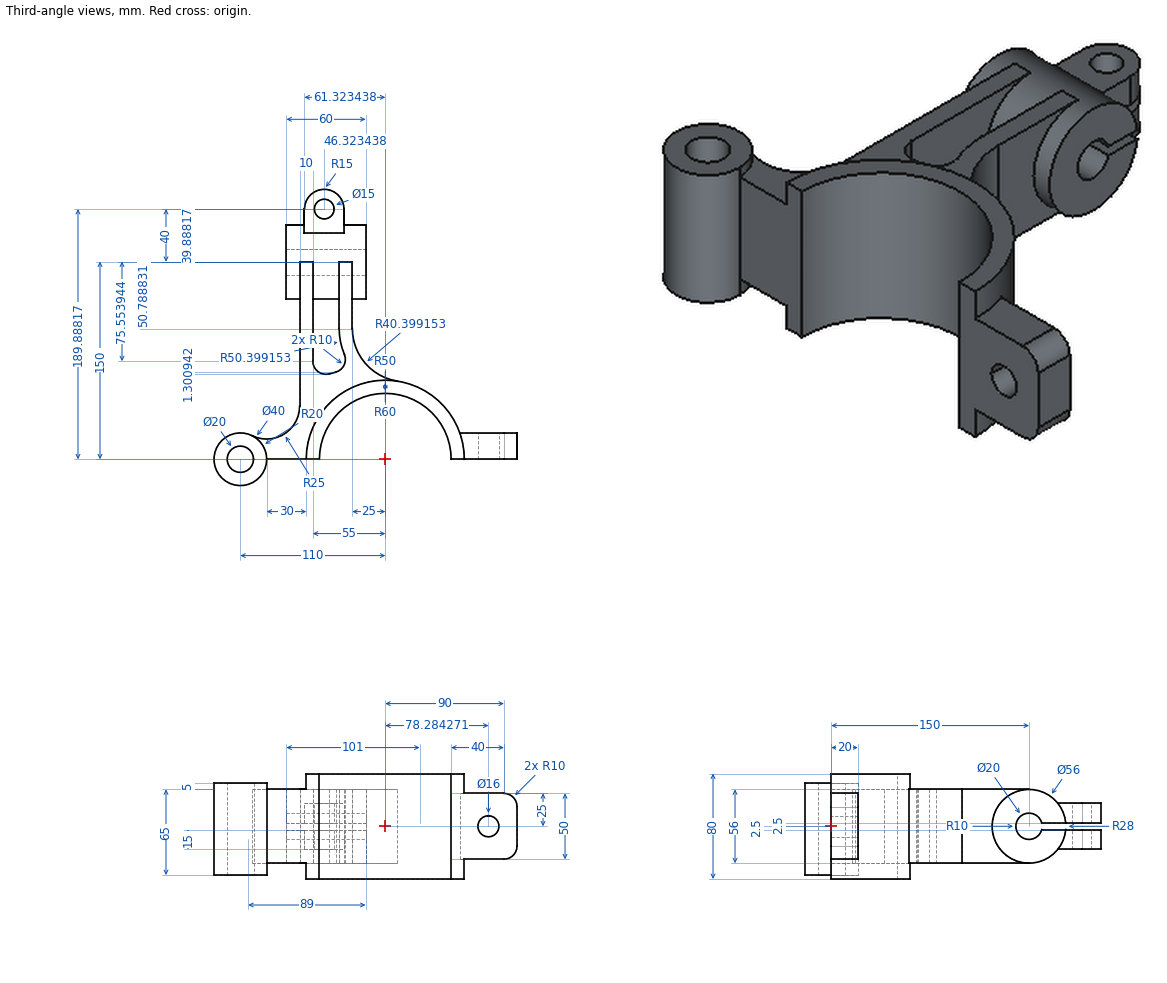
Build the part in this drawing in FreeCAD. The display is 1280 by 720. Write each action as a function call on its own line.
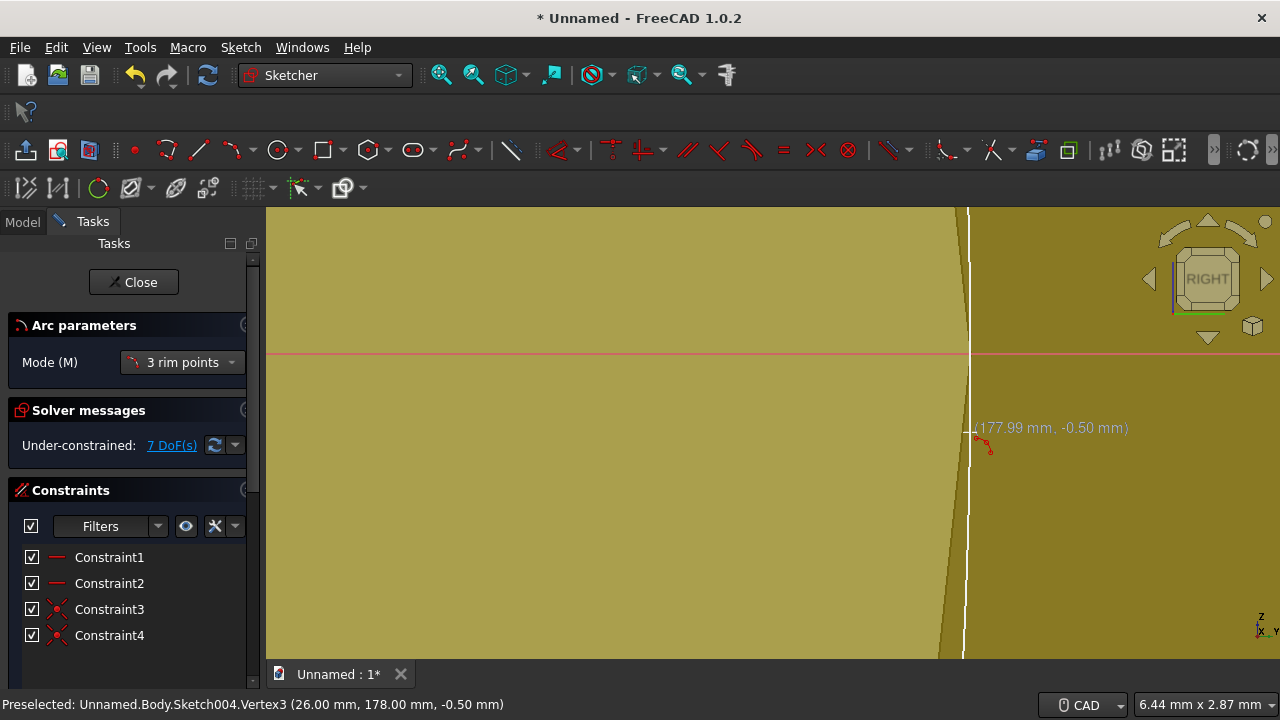
scroll(976, 441, down, 12)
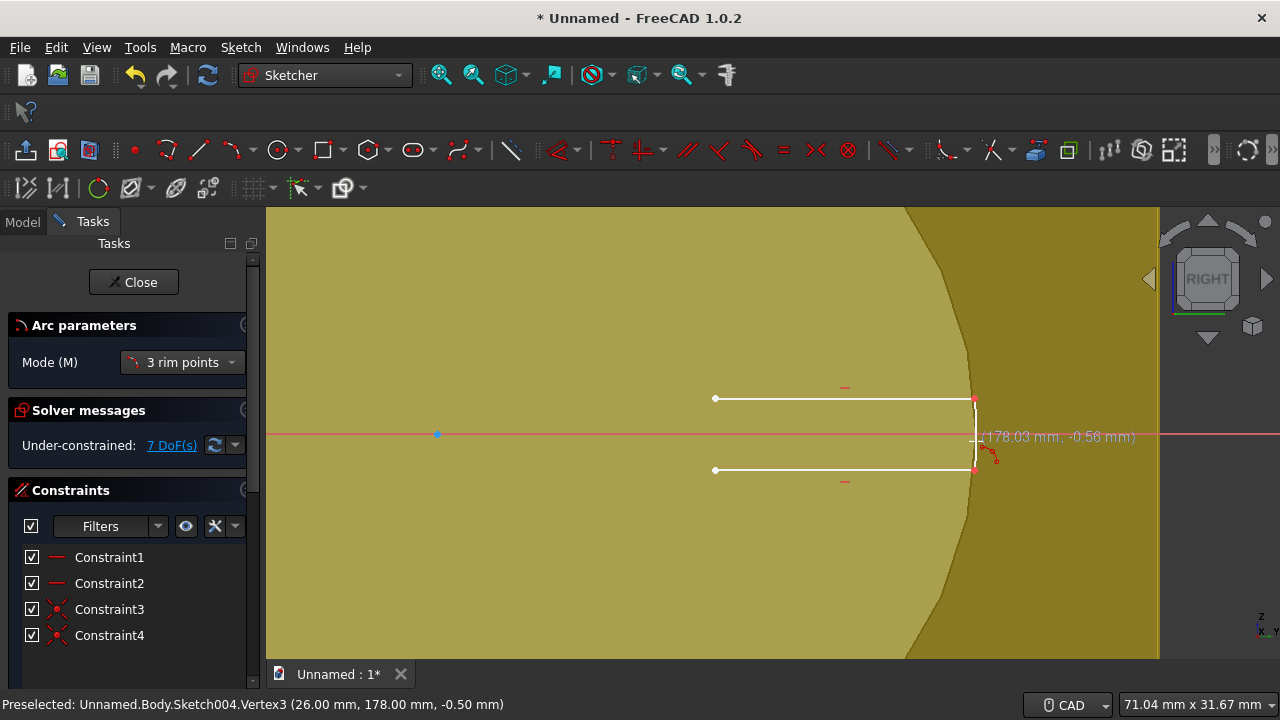
click(715, 470)
click(715, 399)
click(457, 356)
key(Escape)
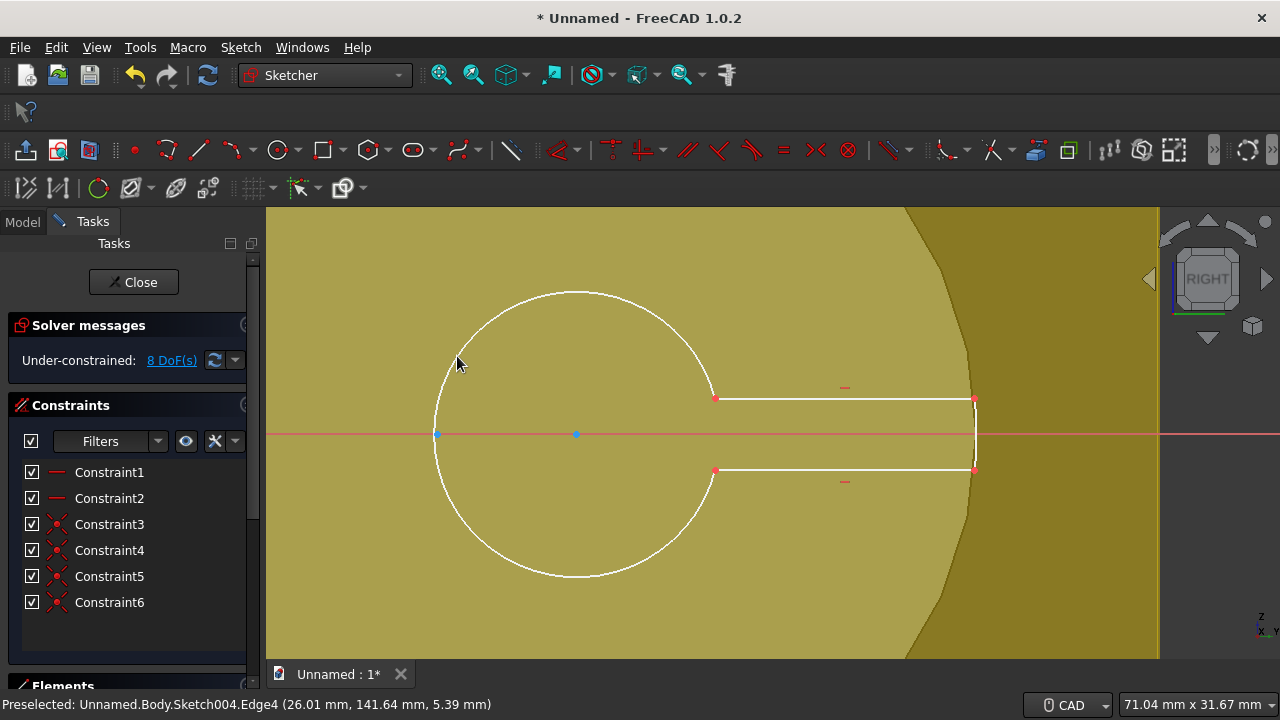
click(976, 449)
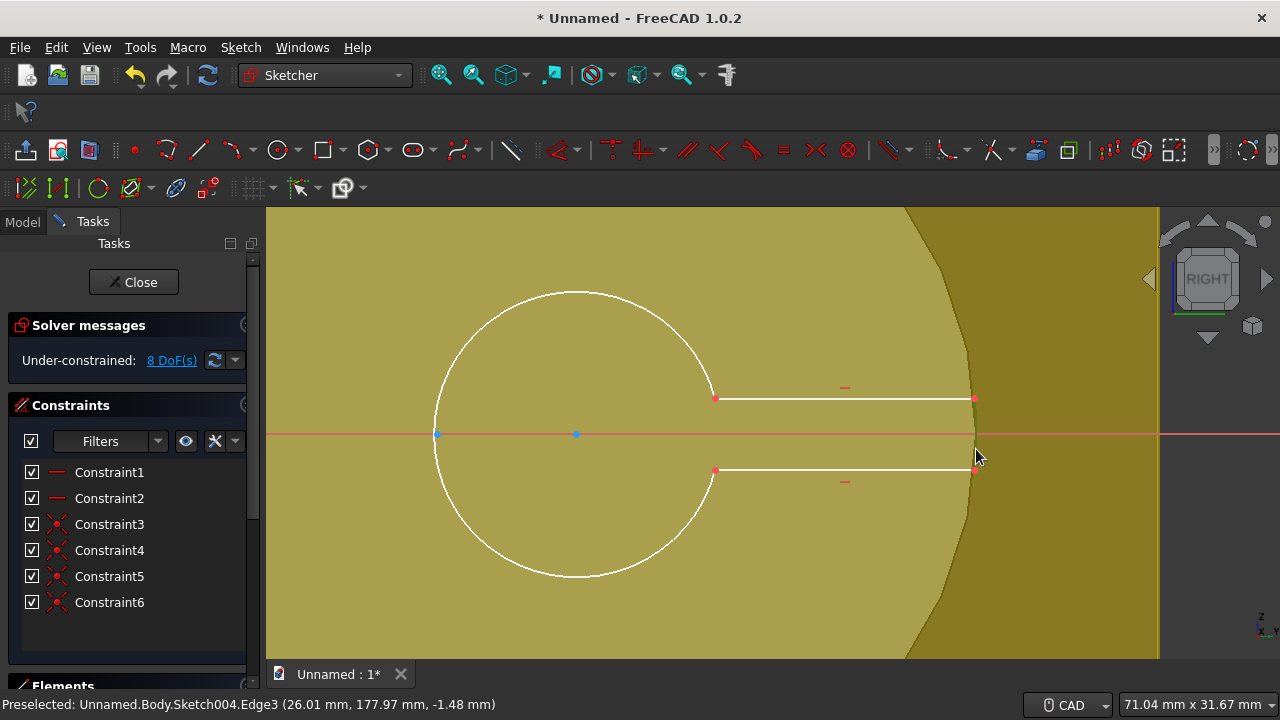
click(519, 304)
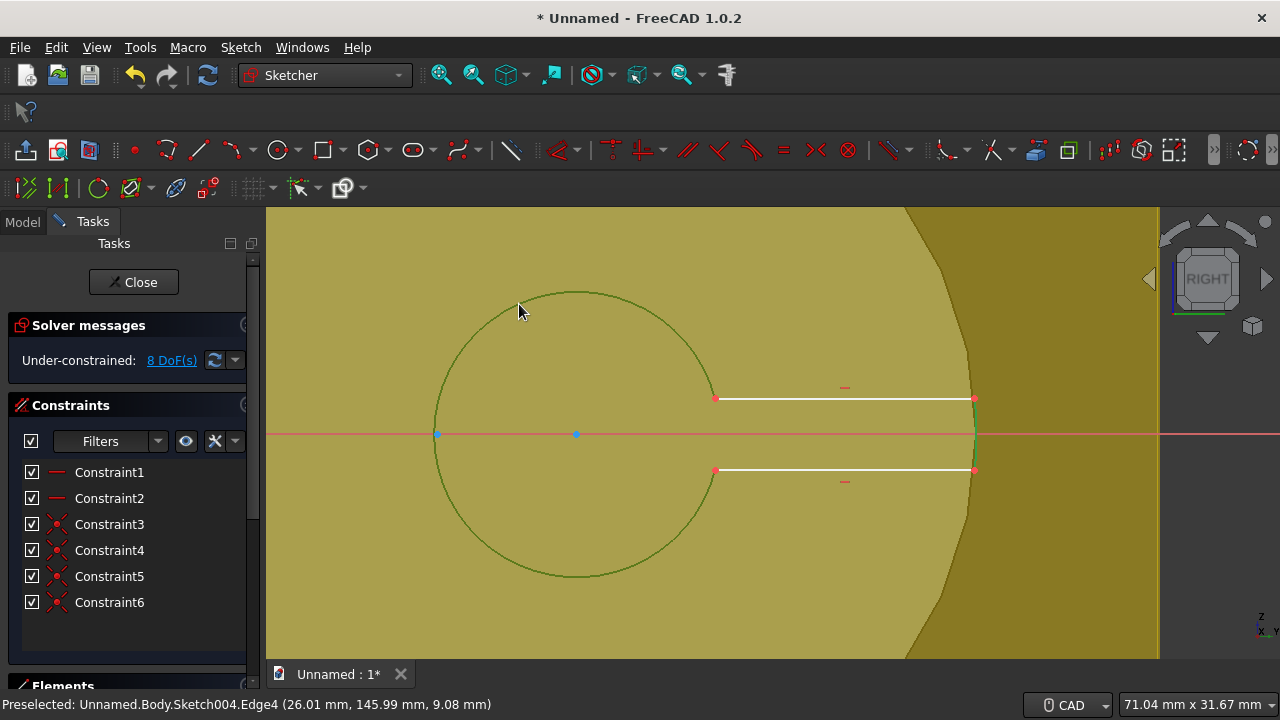
key(c)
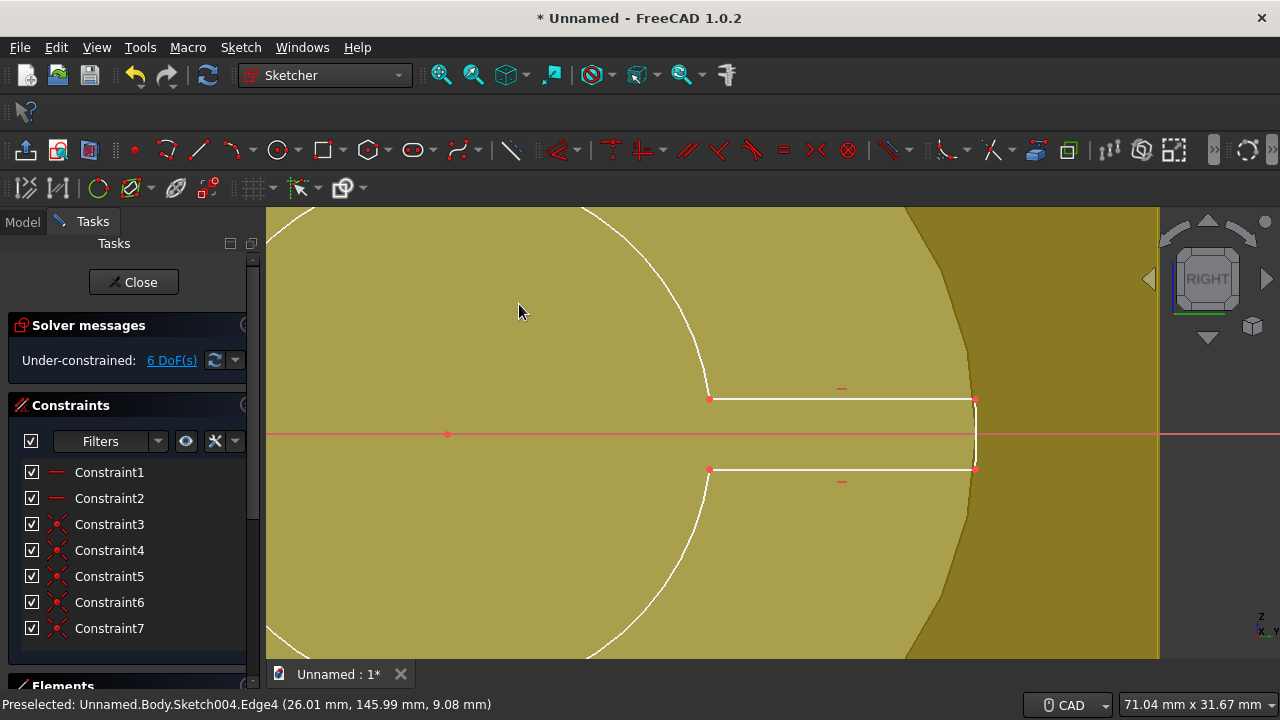
click(448, 435)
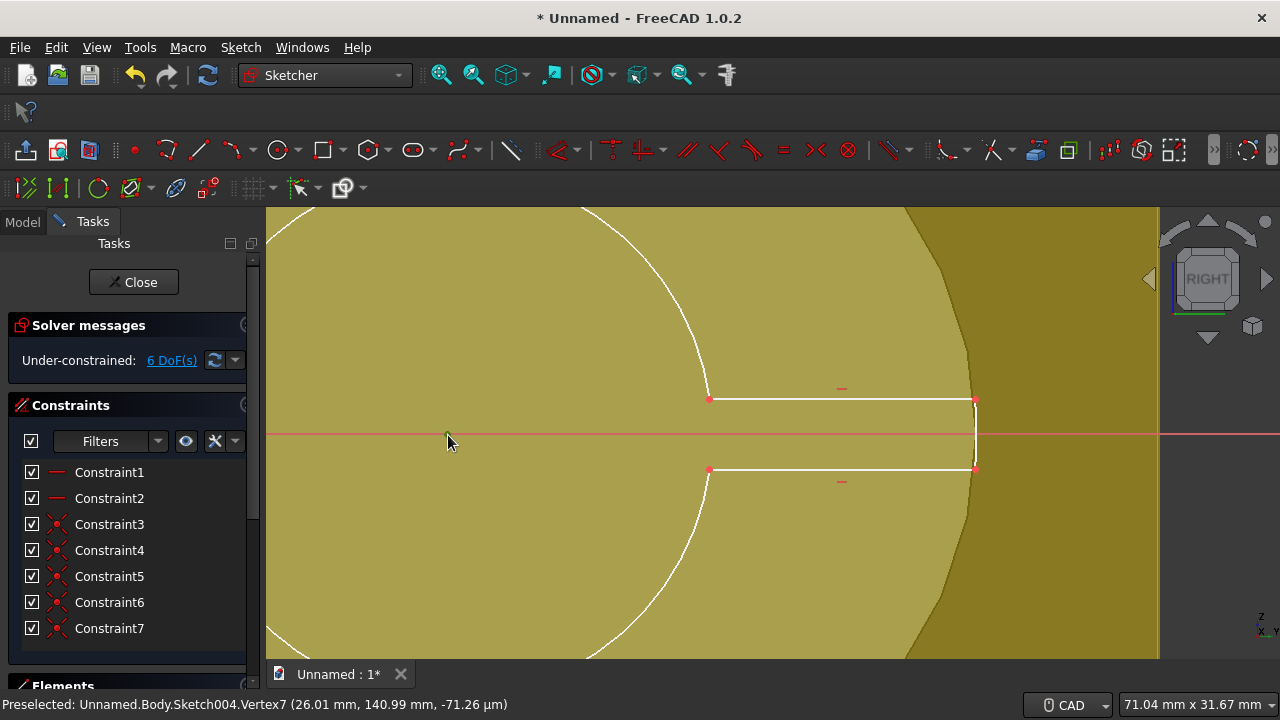
click(353, 434)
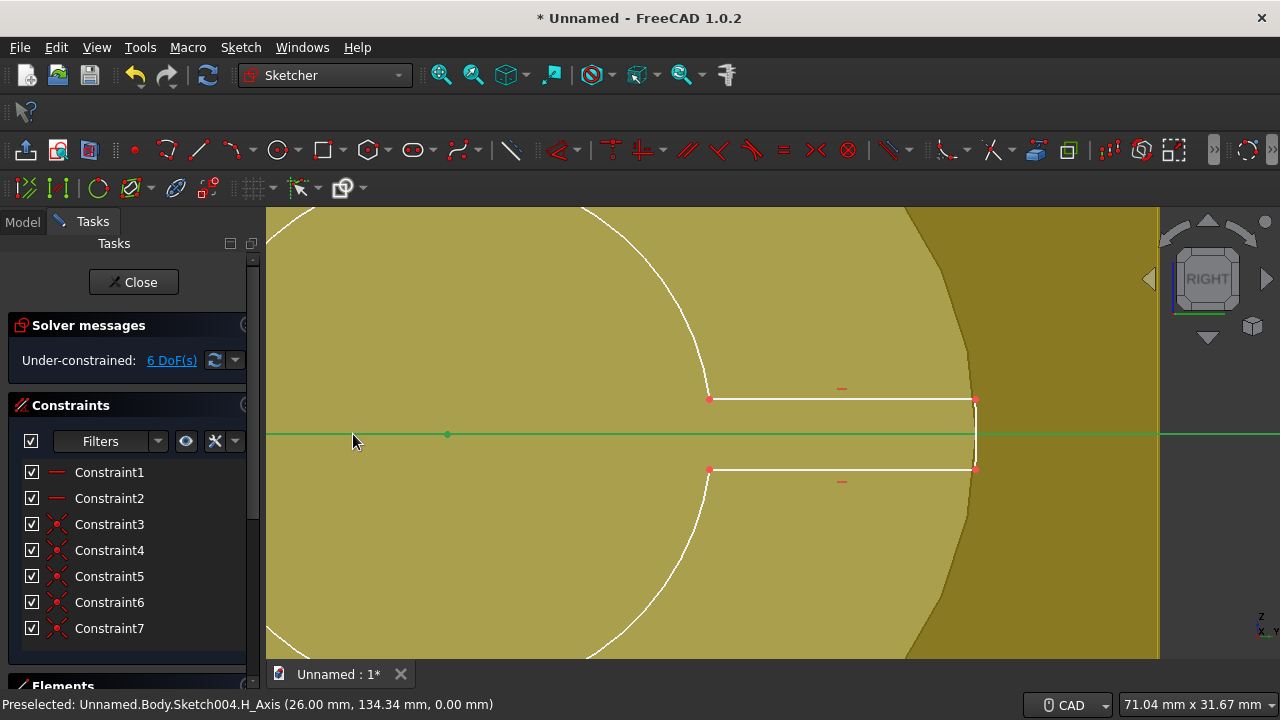
click(612, 150)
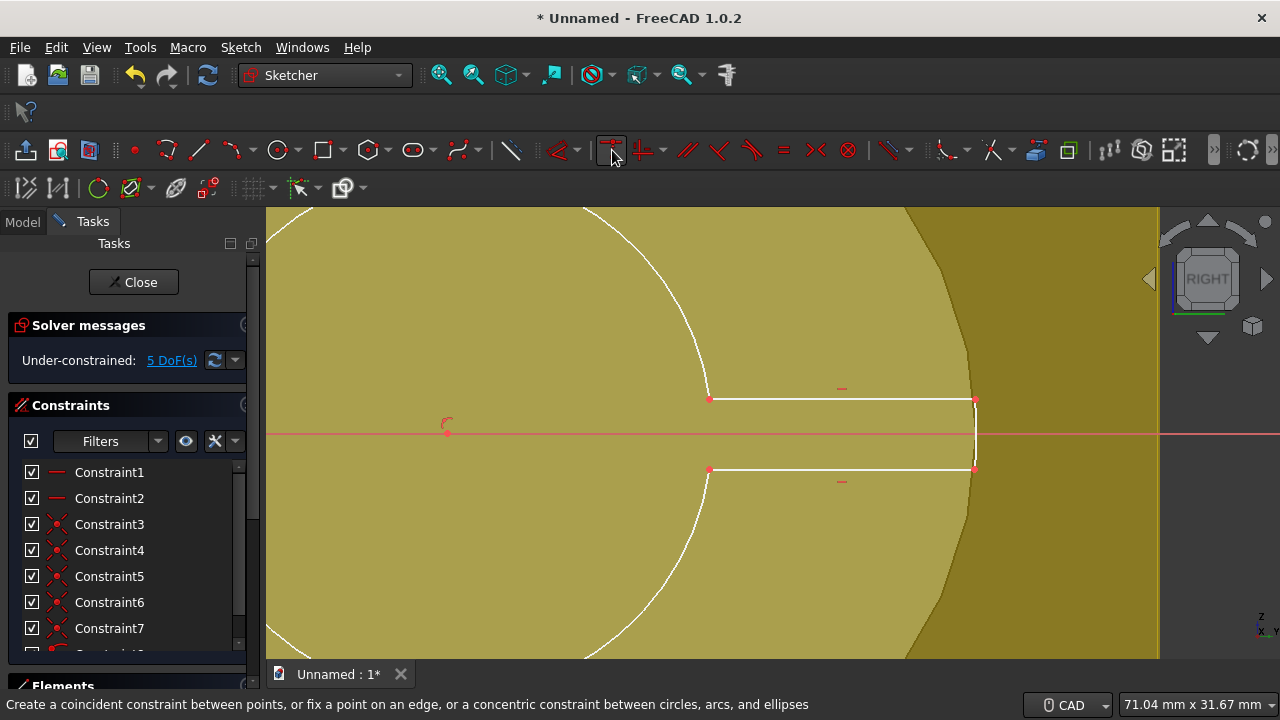
key(d)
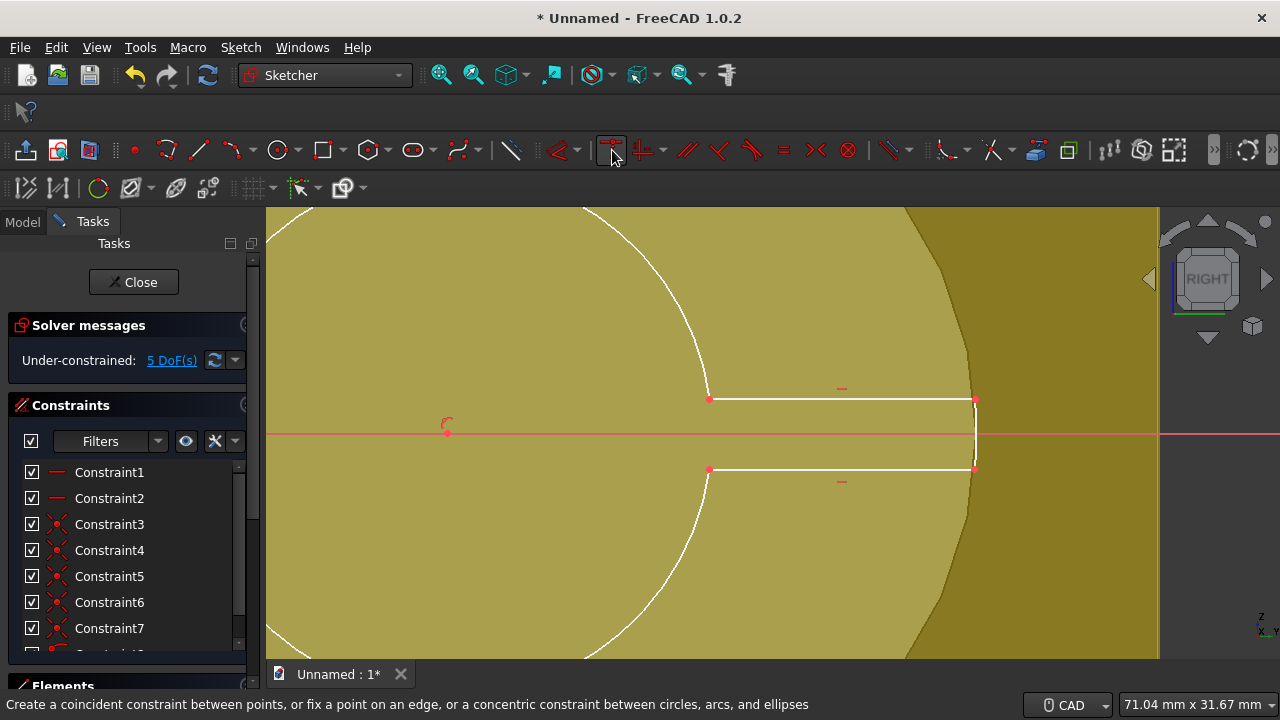
click(976, 449)
click(1008, 450)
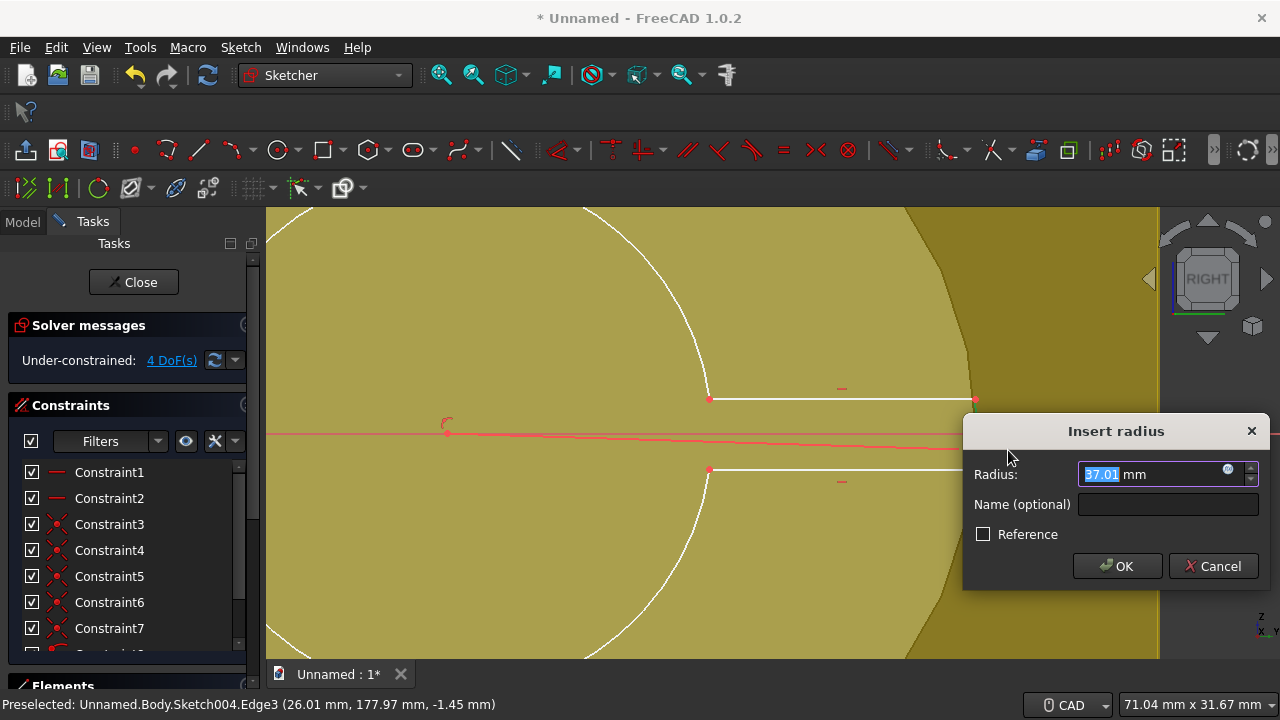
text(28)
key(Return)